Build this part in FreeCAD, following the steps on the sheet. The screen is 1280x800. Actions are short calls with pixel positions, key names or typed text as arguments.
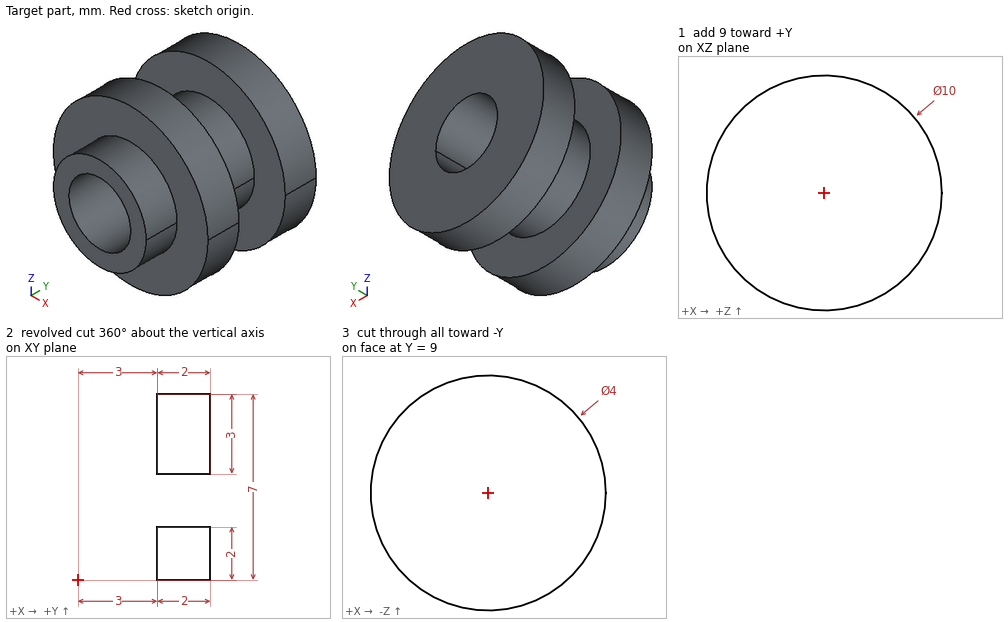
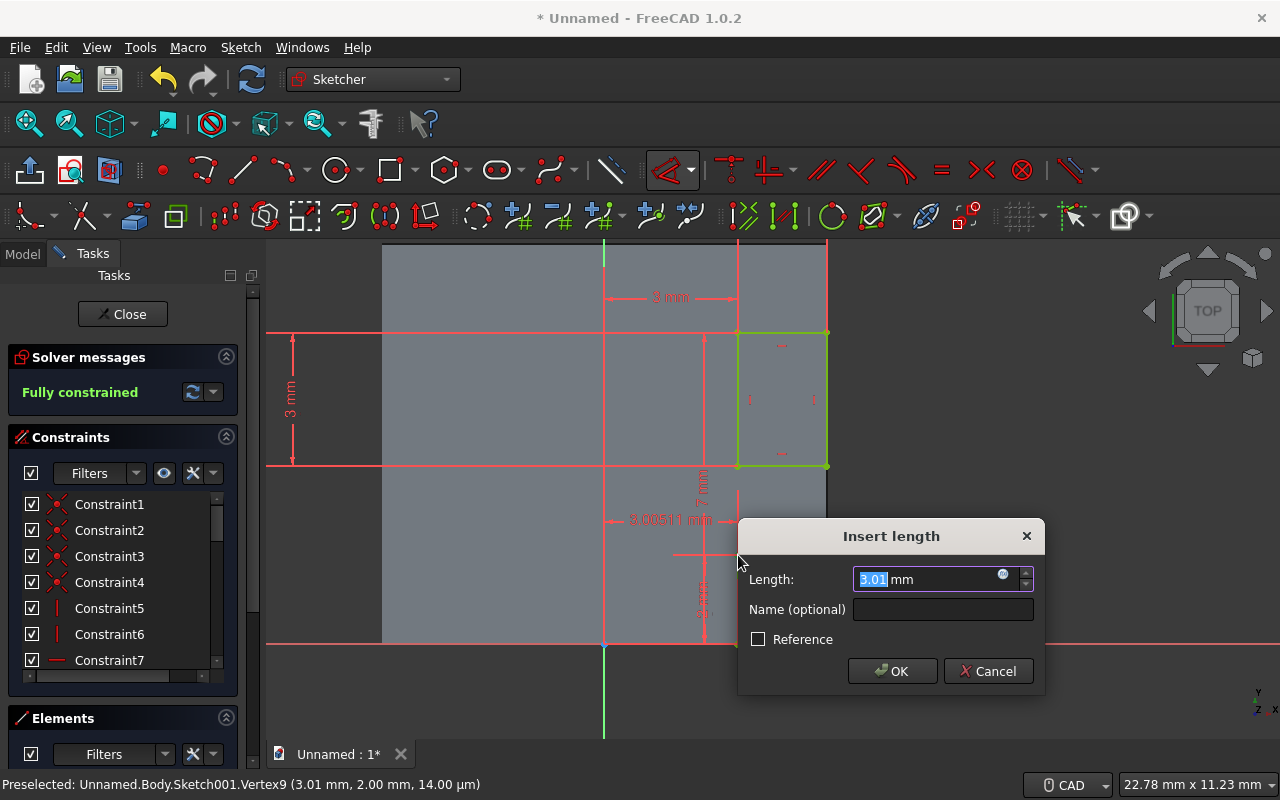
text(3)
key(Return)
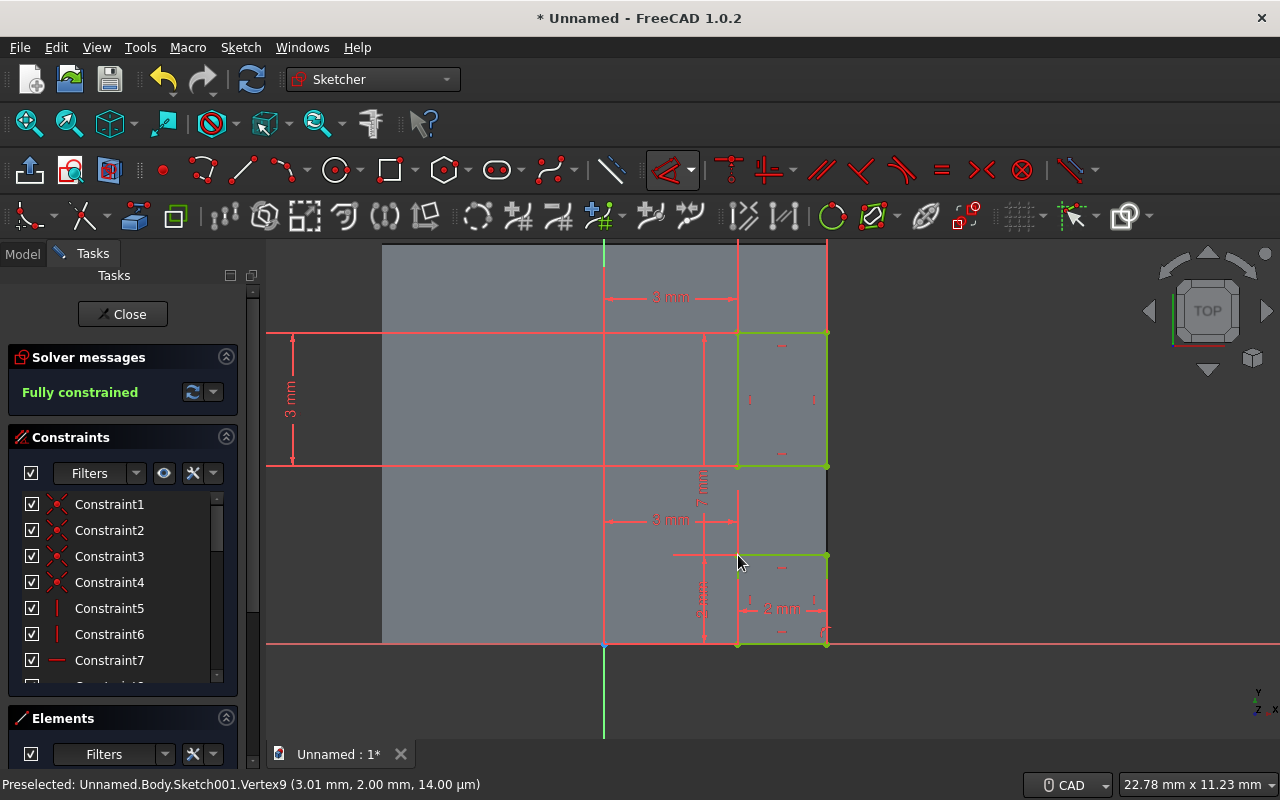
click(123, 314)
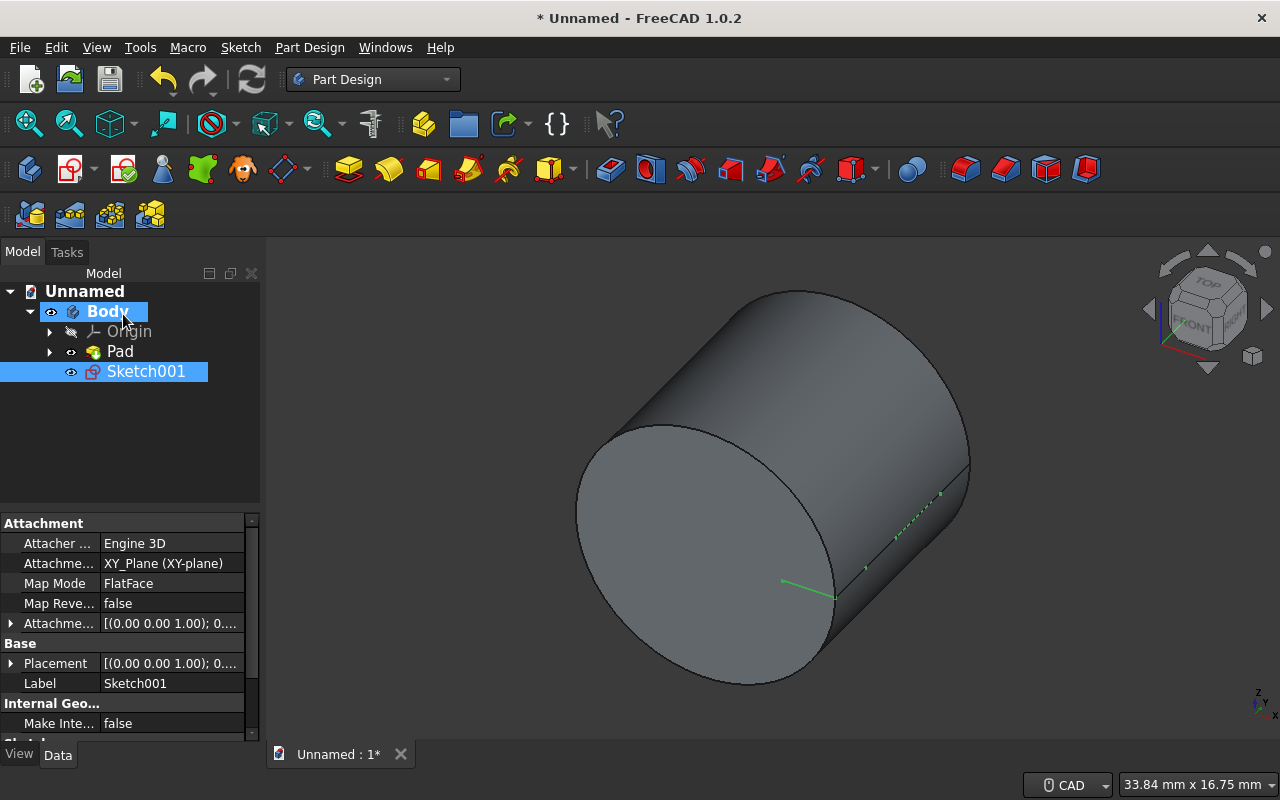
click(692, 170)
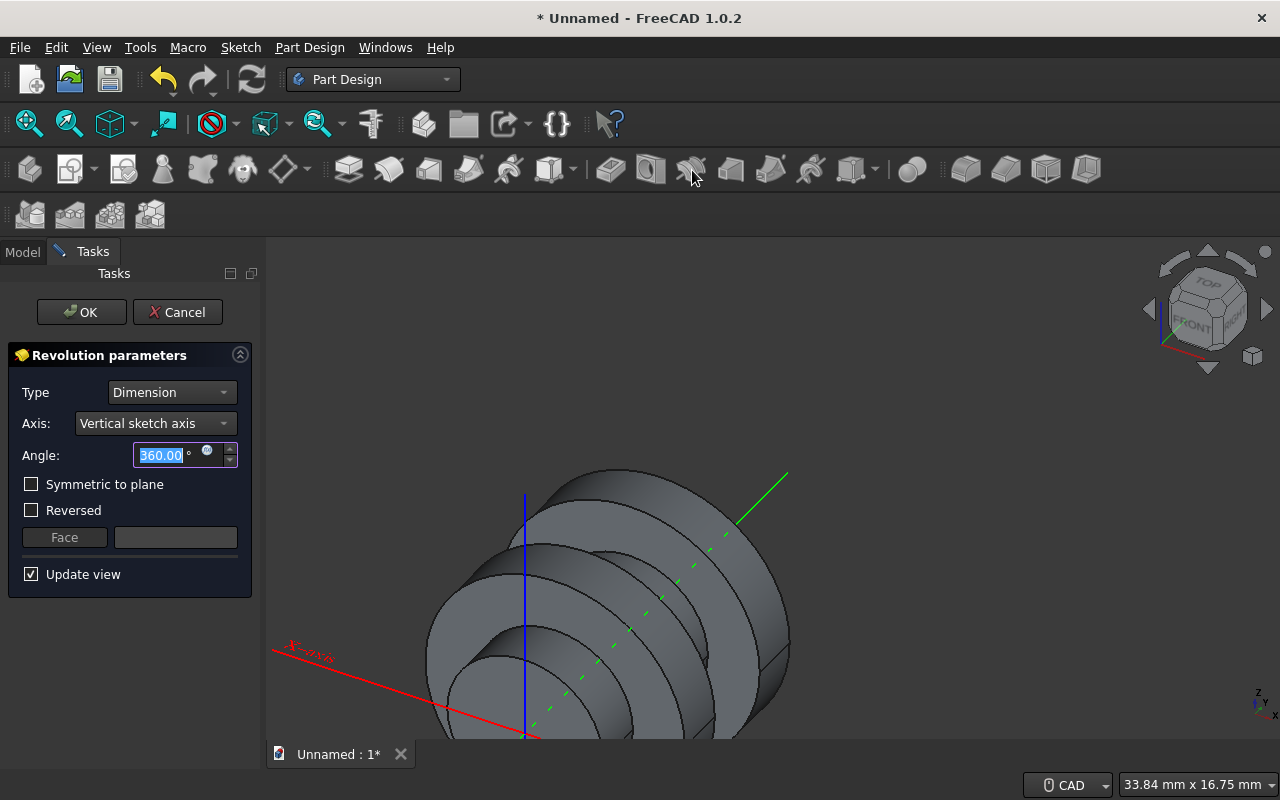
click(82, 312)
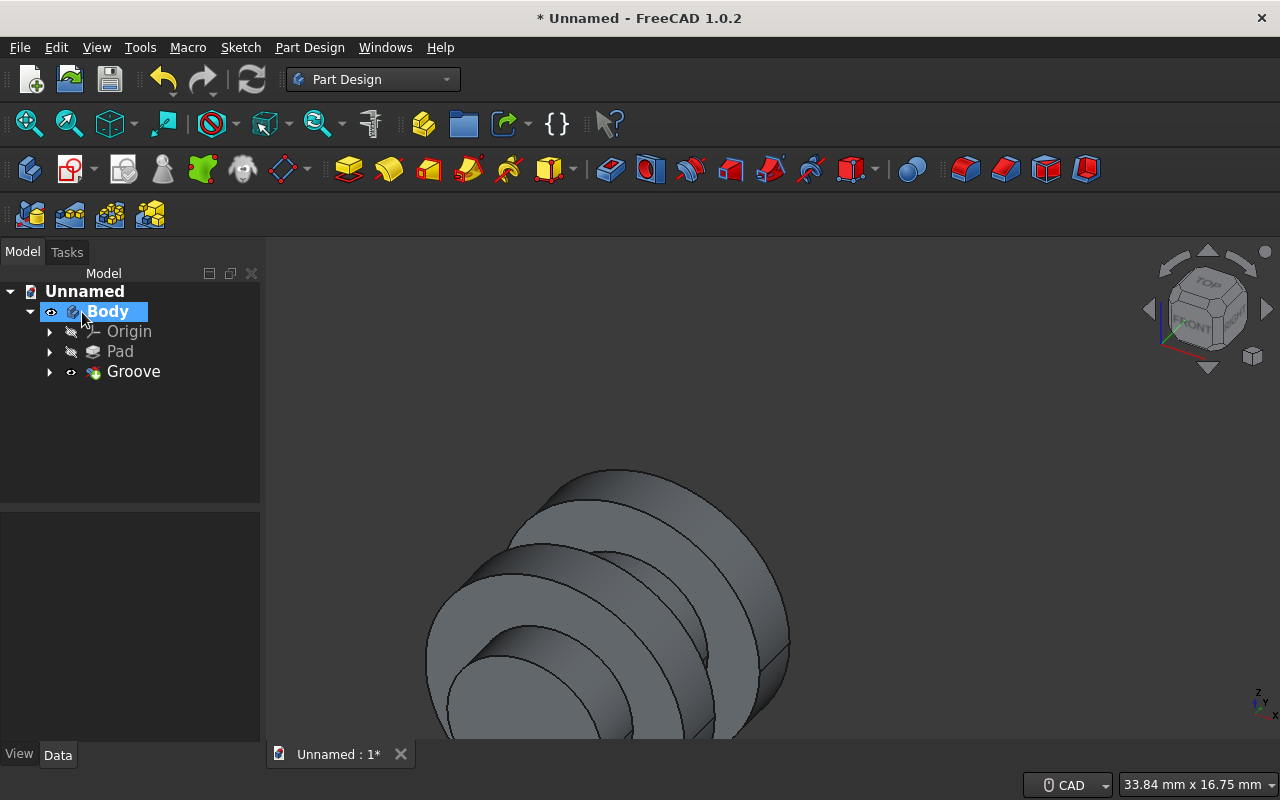
click(30, 124)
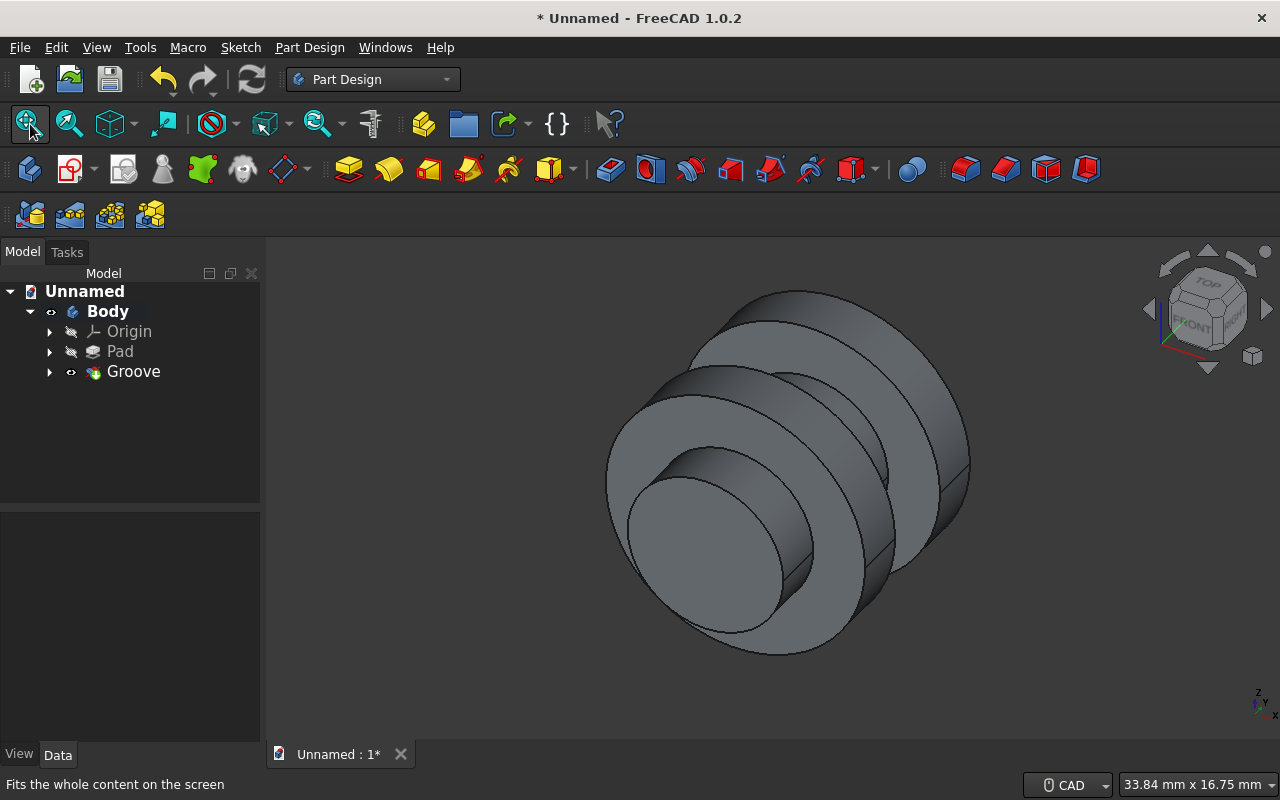
key(4)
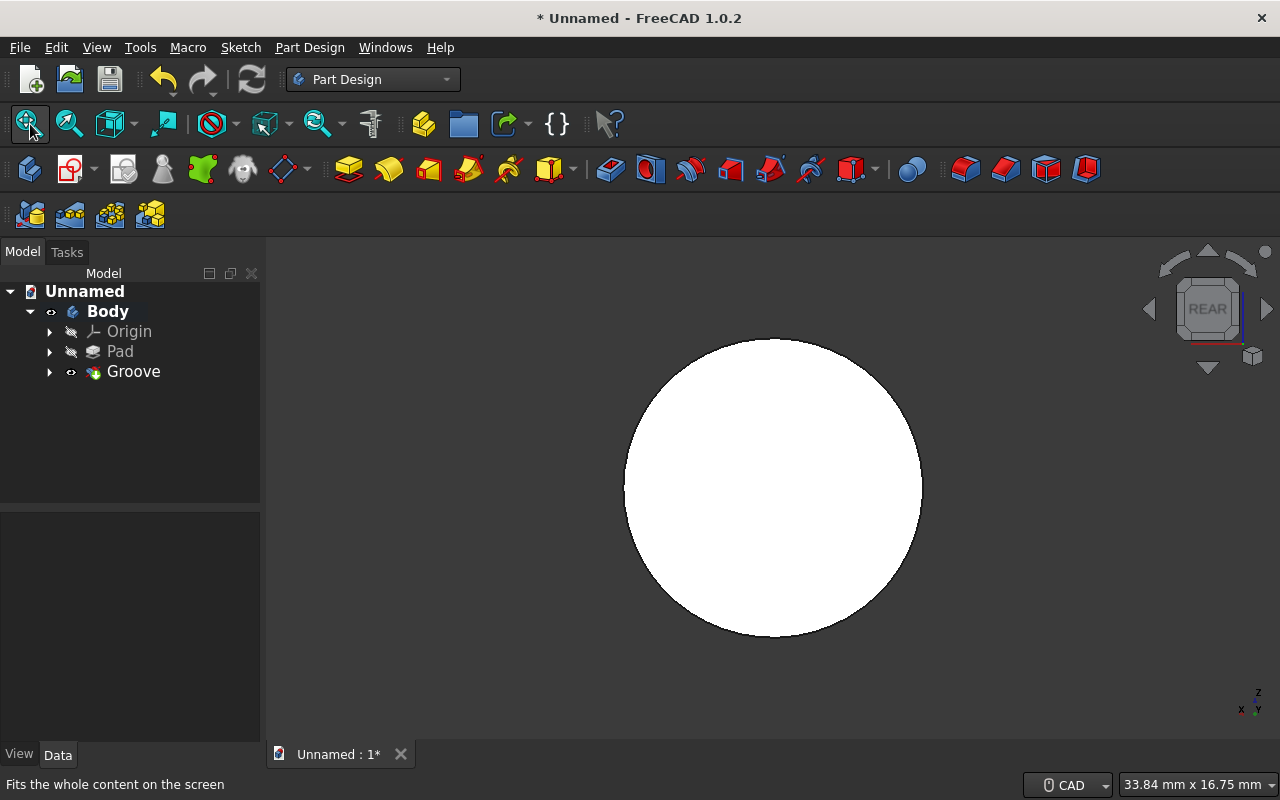
click(773, 487)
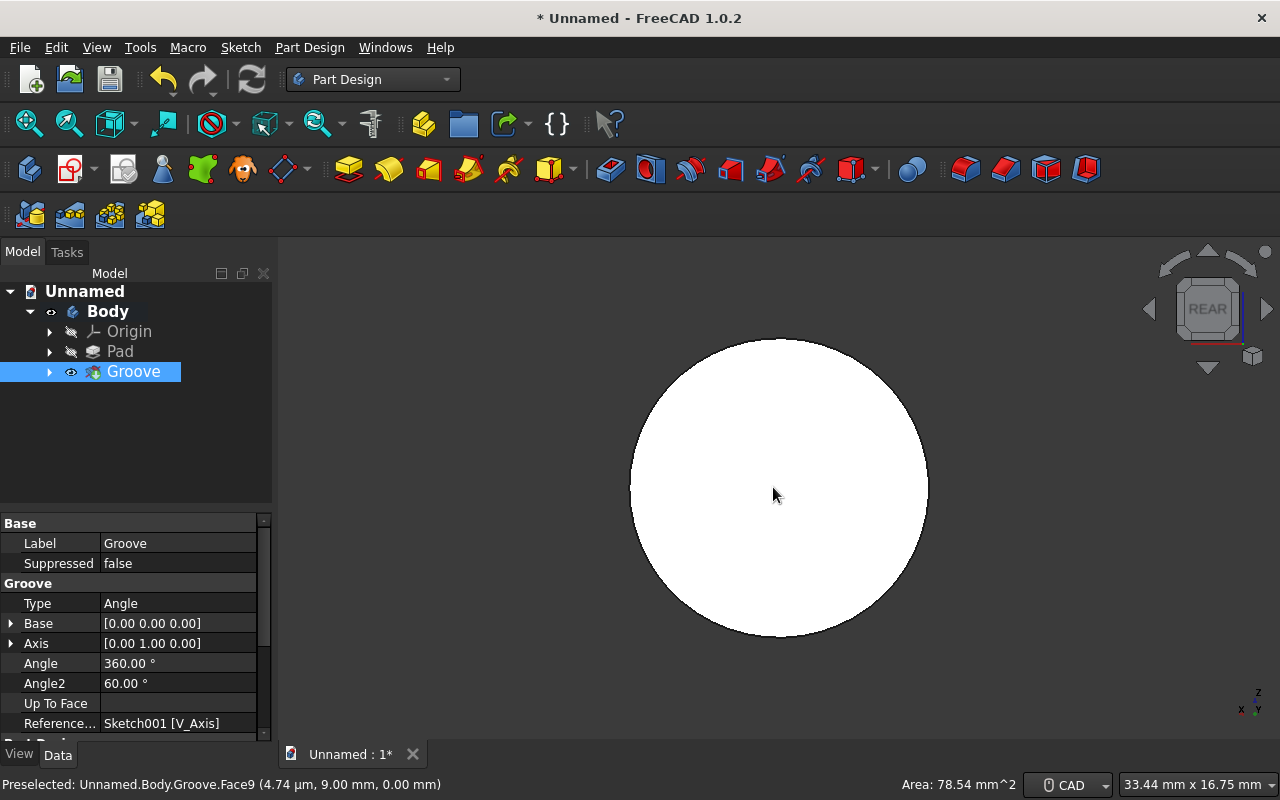
click(70, 170)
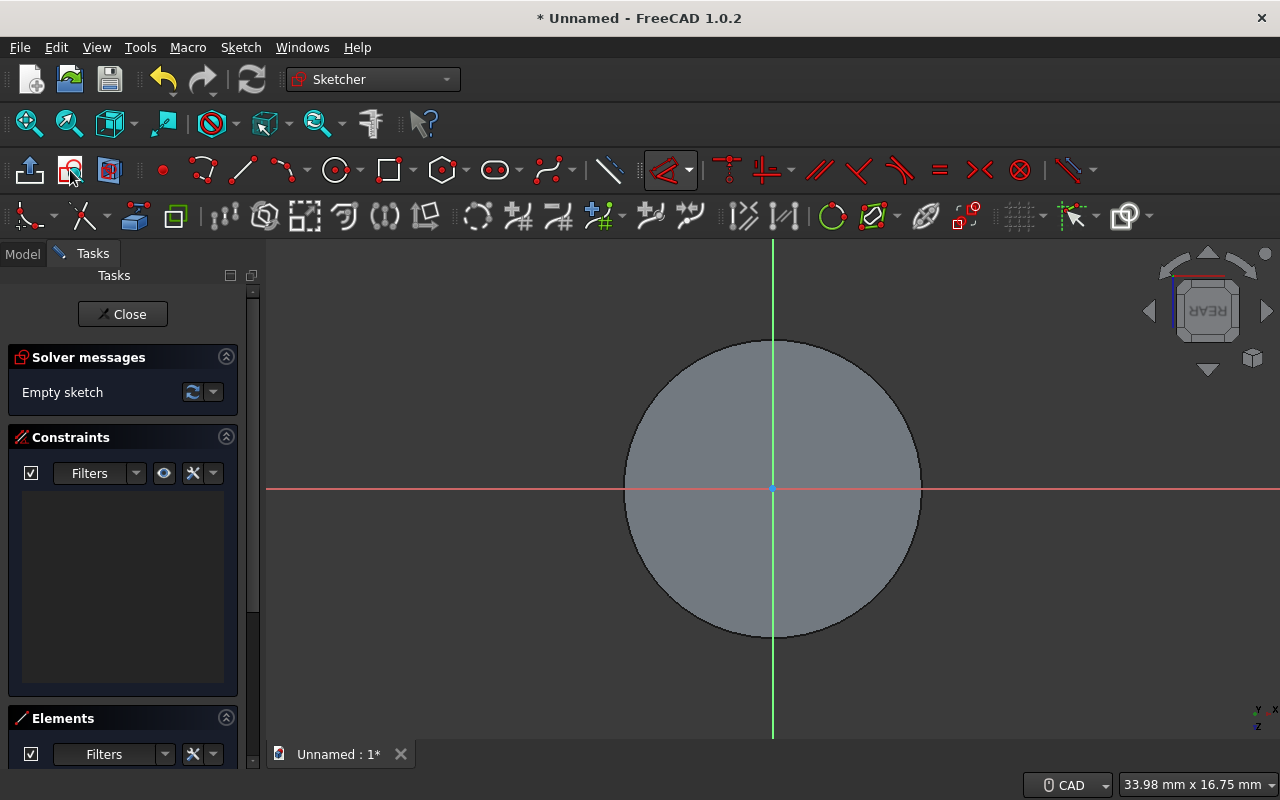
scroll(813, 489, up, 5)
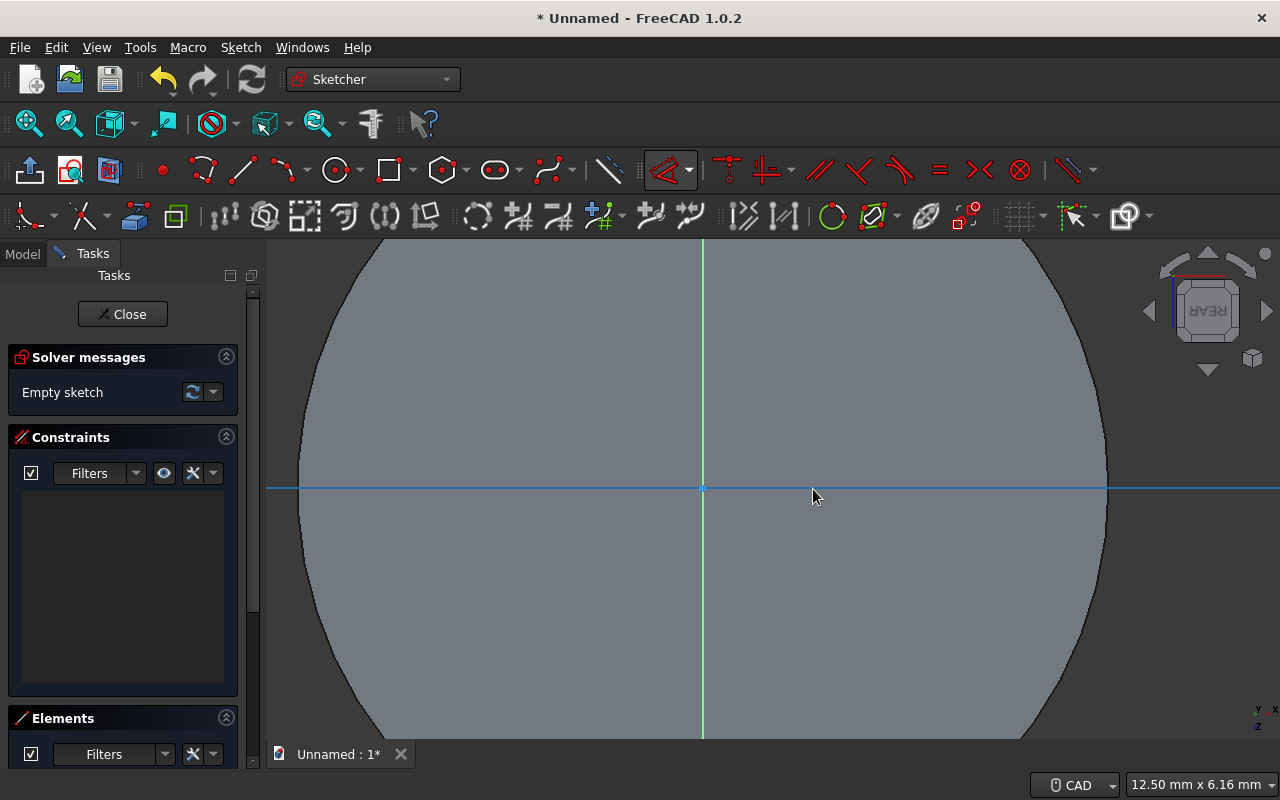
click(336, 170)